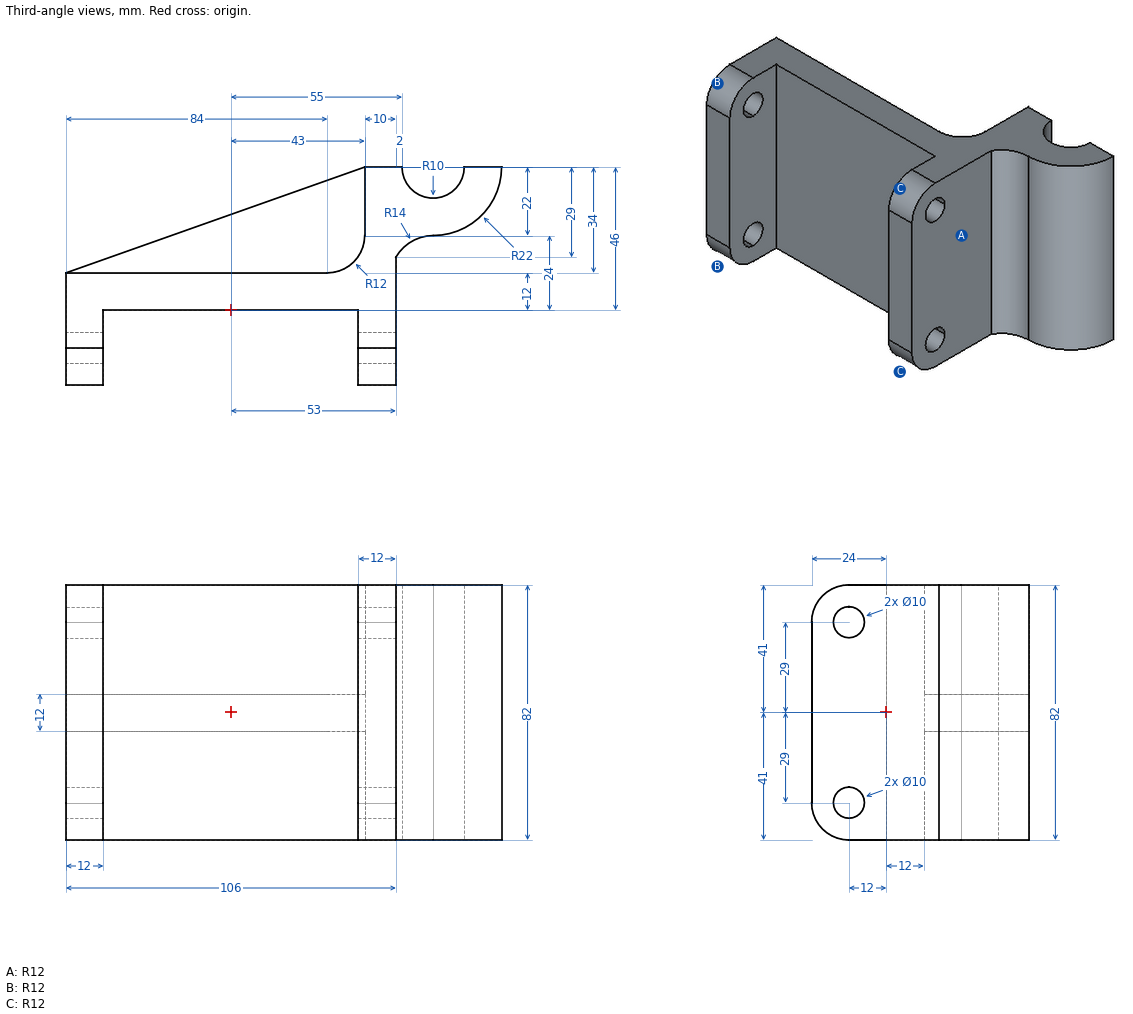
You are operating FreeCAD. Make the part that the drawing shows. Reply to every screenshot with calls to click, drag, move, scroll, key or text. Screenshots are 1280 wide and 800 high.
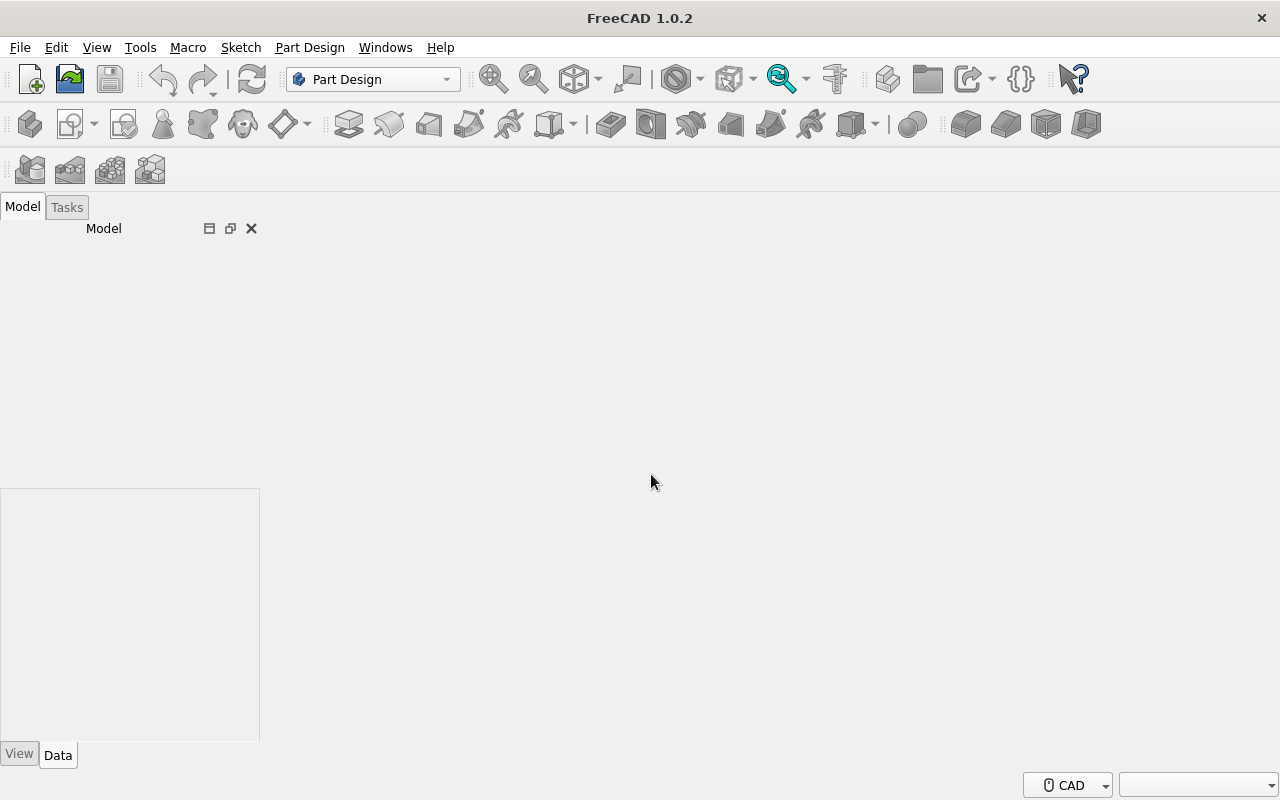
click(30, 80)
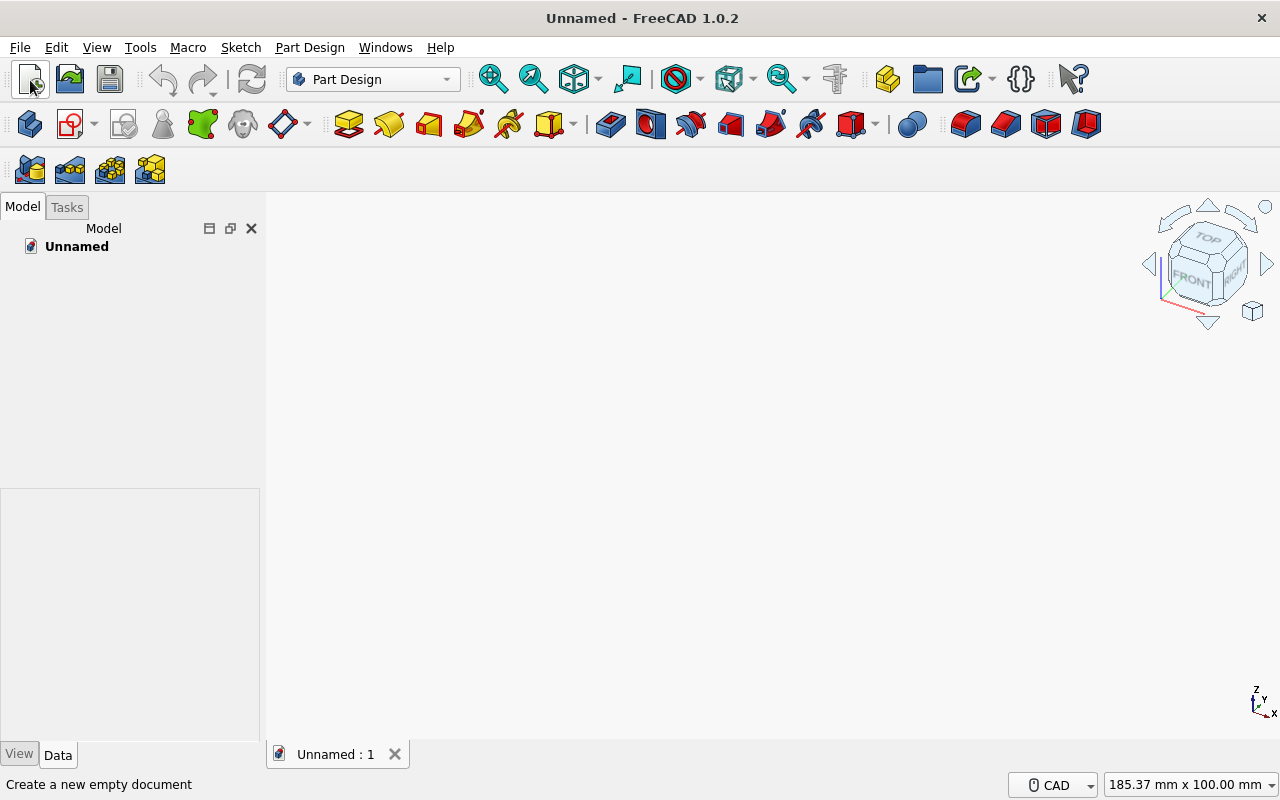
click(70, 124)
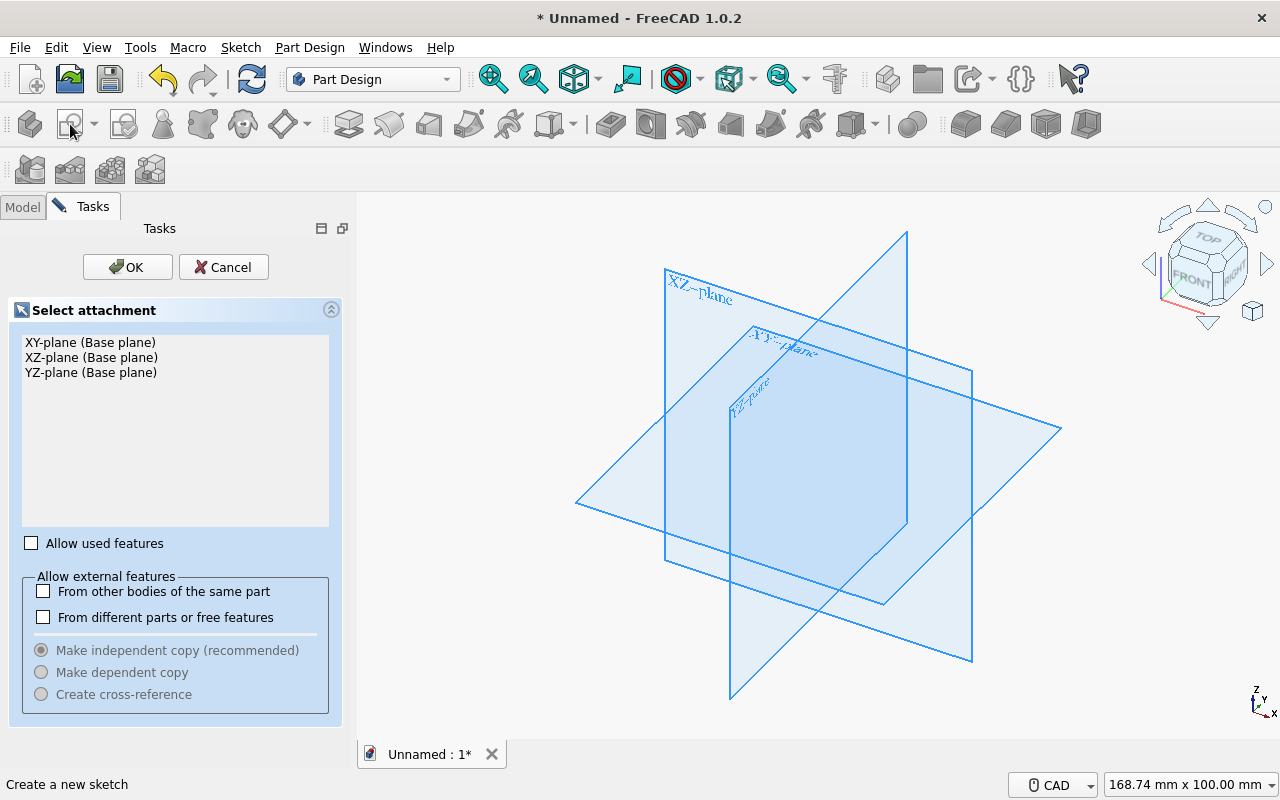
click(82, 358)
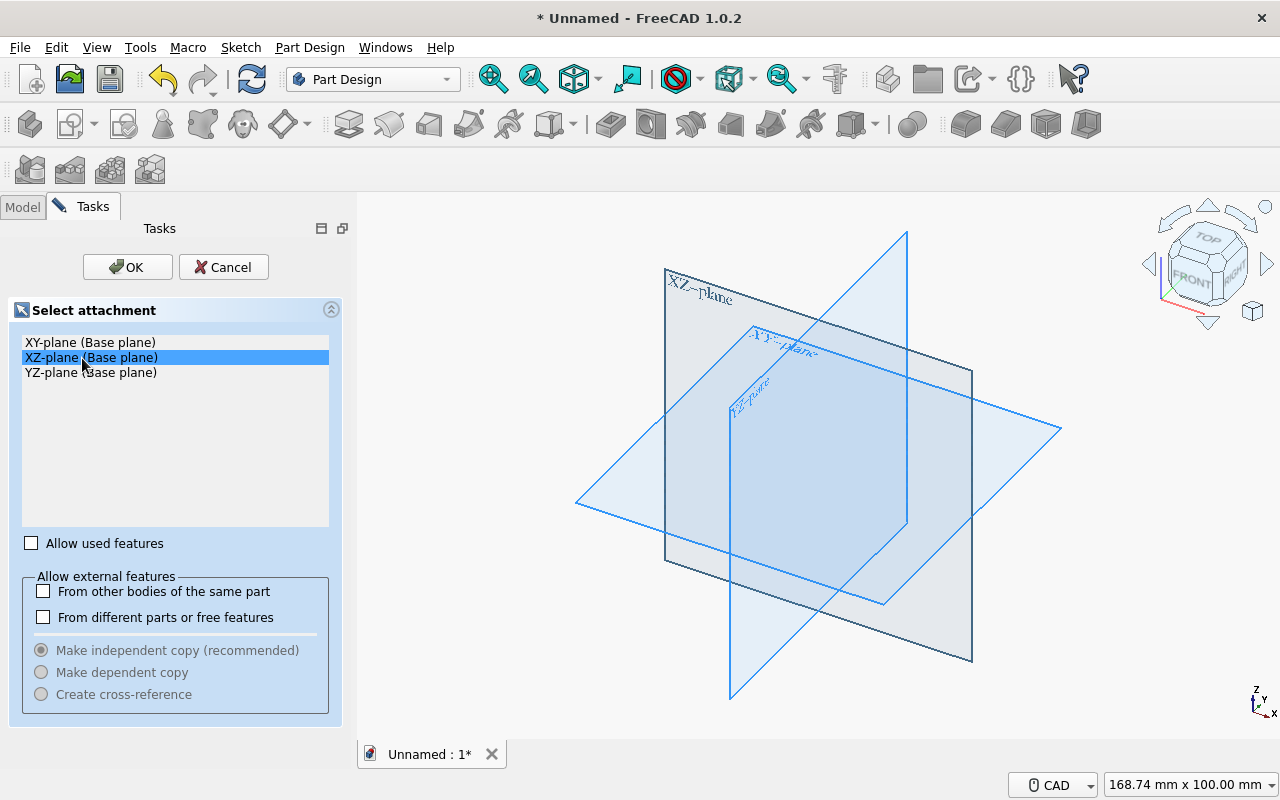
click(128, 267)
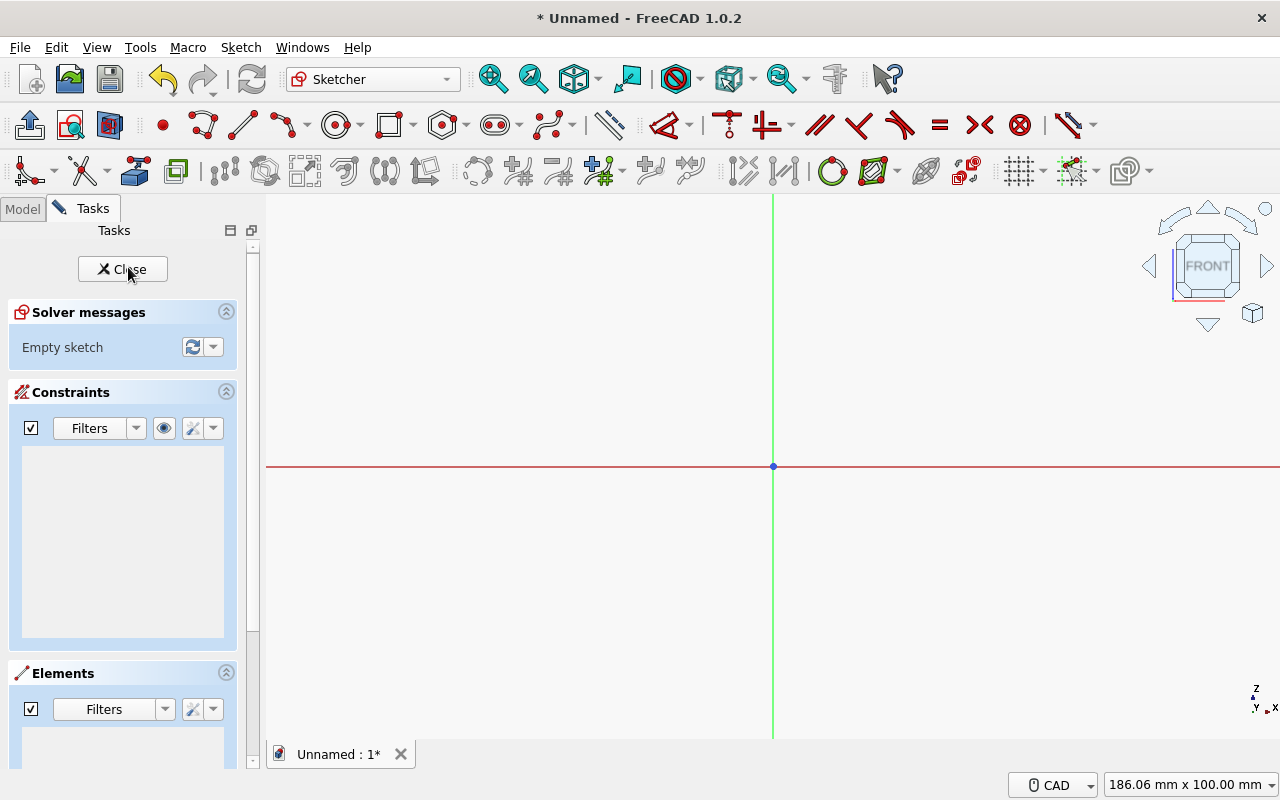
scroll(395, 467, down, 1)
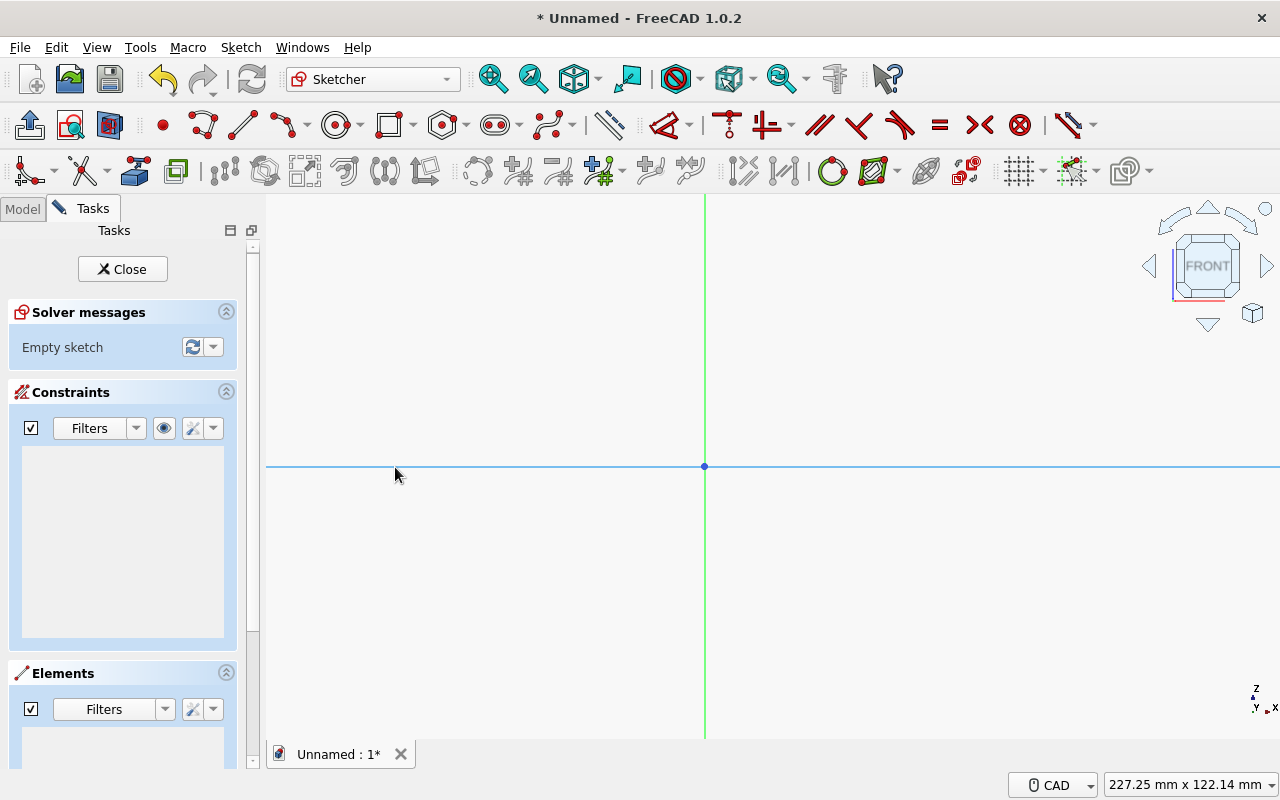
key(g)
key(v)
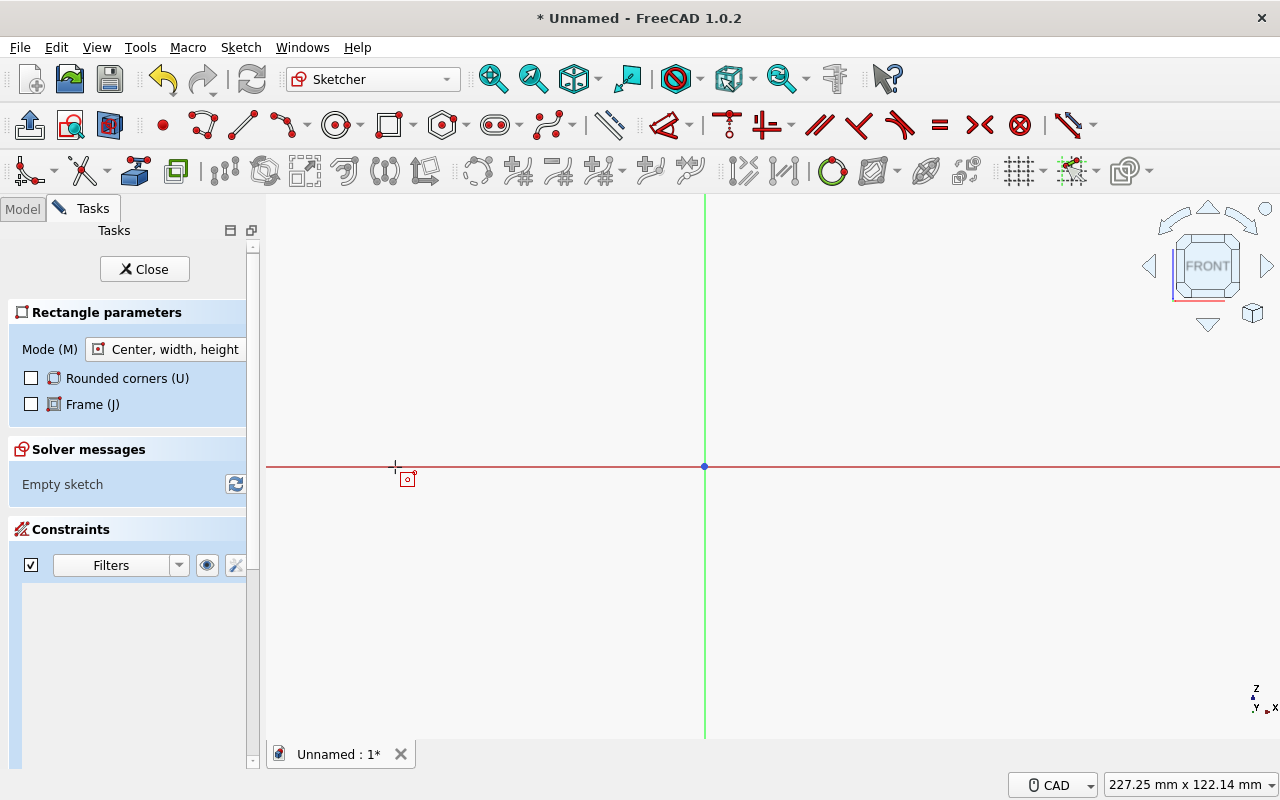
click(705, 467)
move(941, 284)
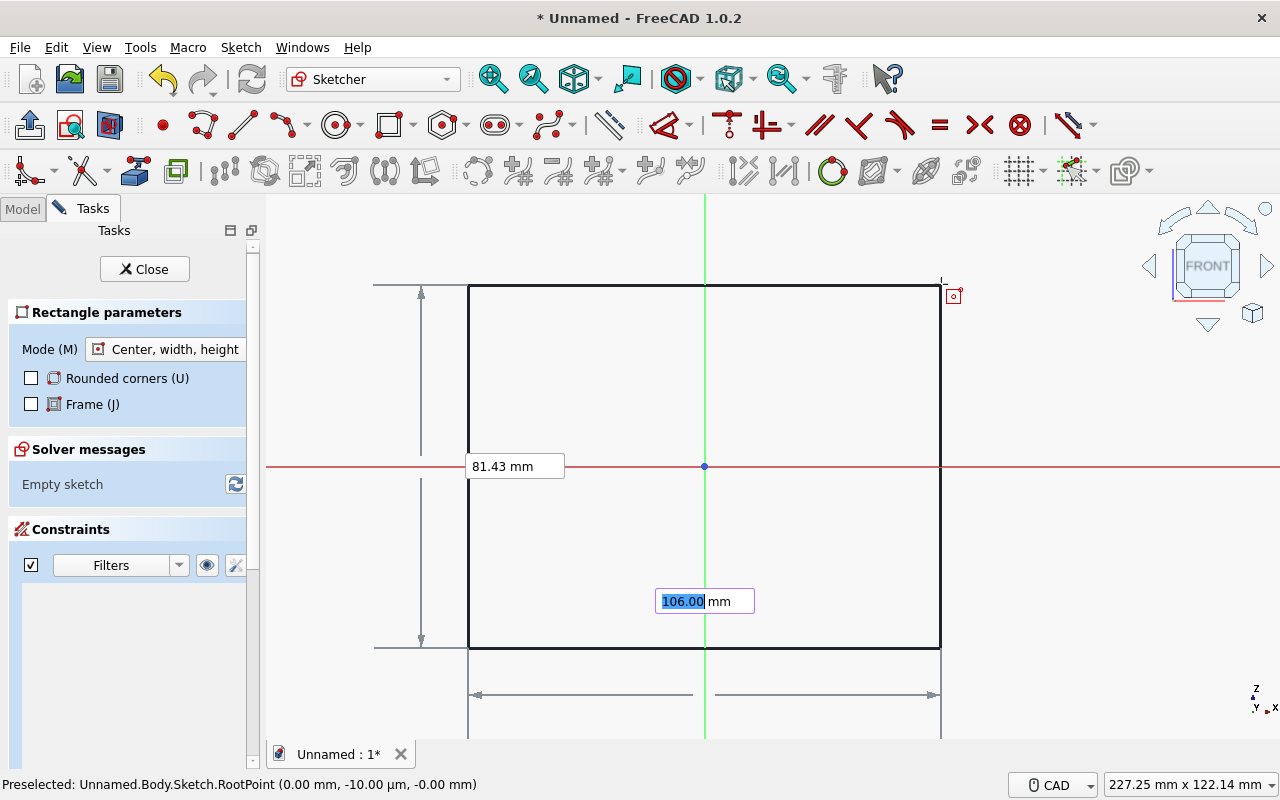
text(106)
key(Tab)
text(82)
key(Return)
key(Escape)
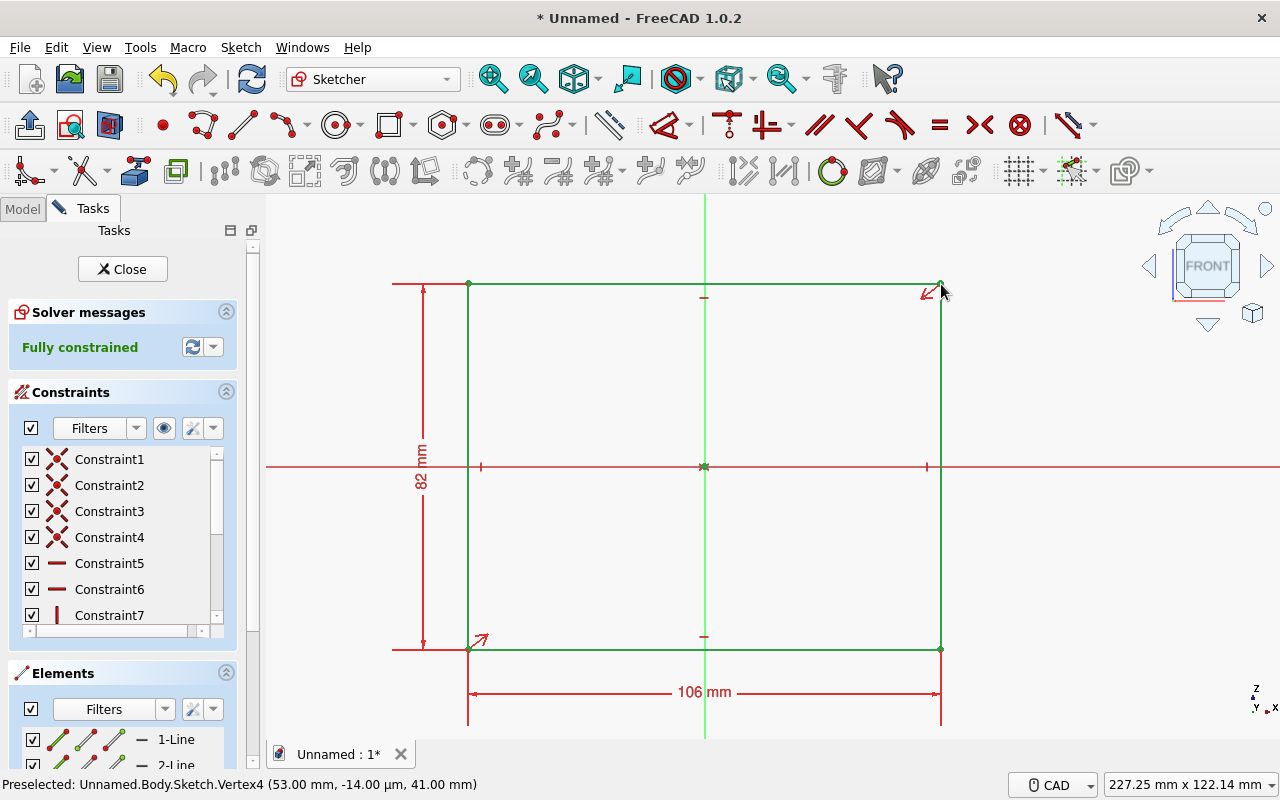
click(123, 269)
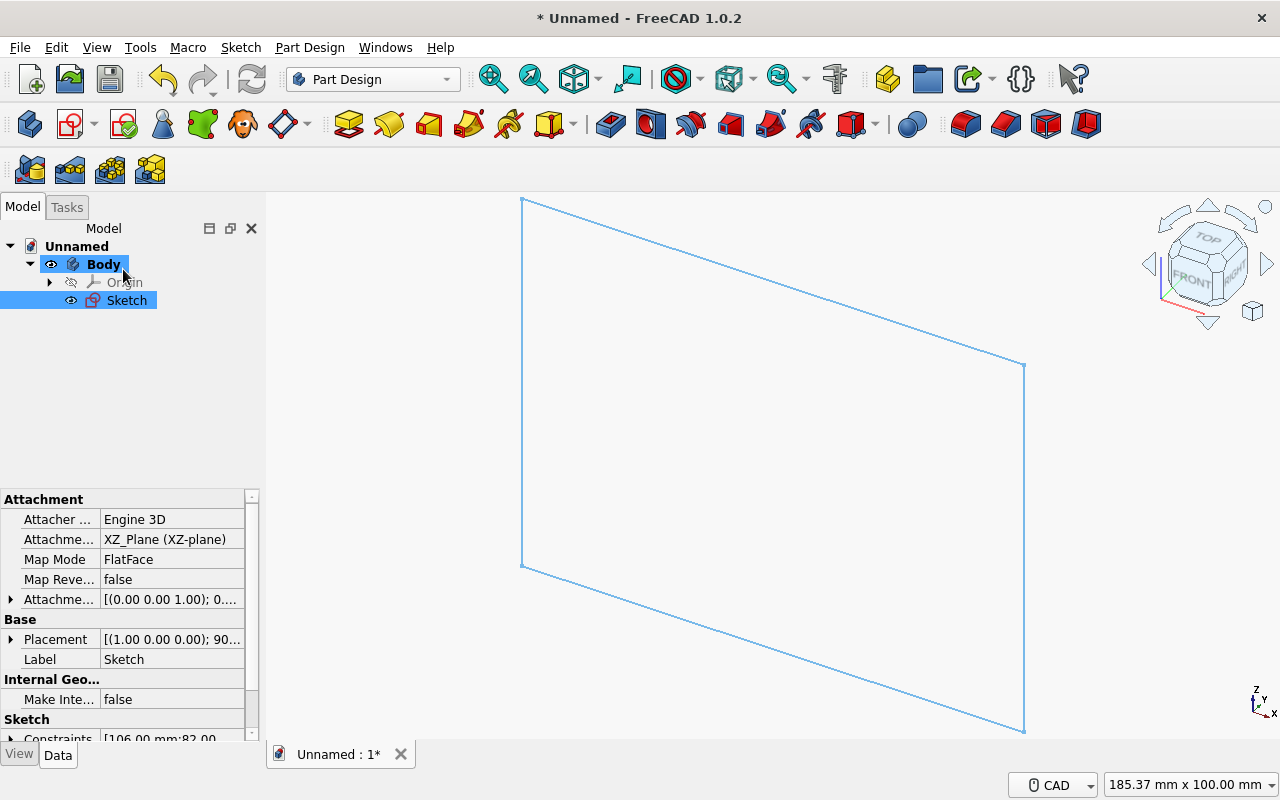
click(350, 124)